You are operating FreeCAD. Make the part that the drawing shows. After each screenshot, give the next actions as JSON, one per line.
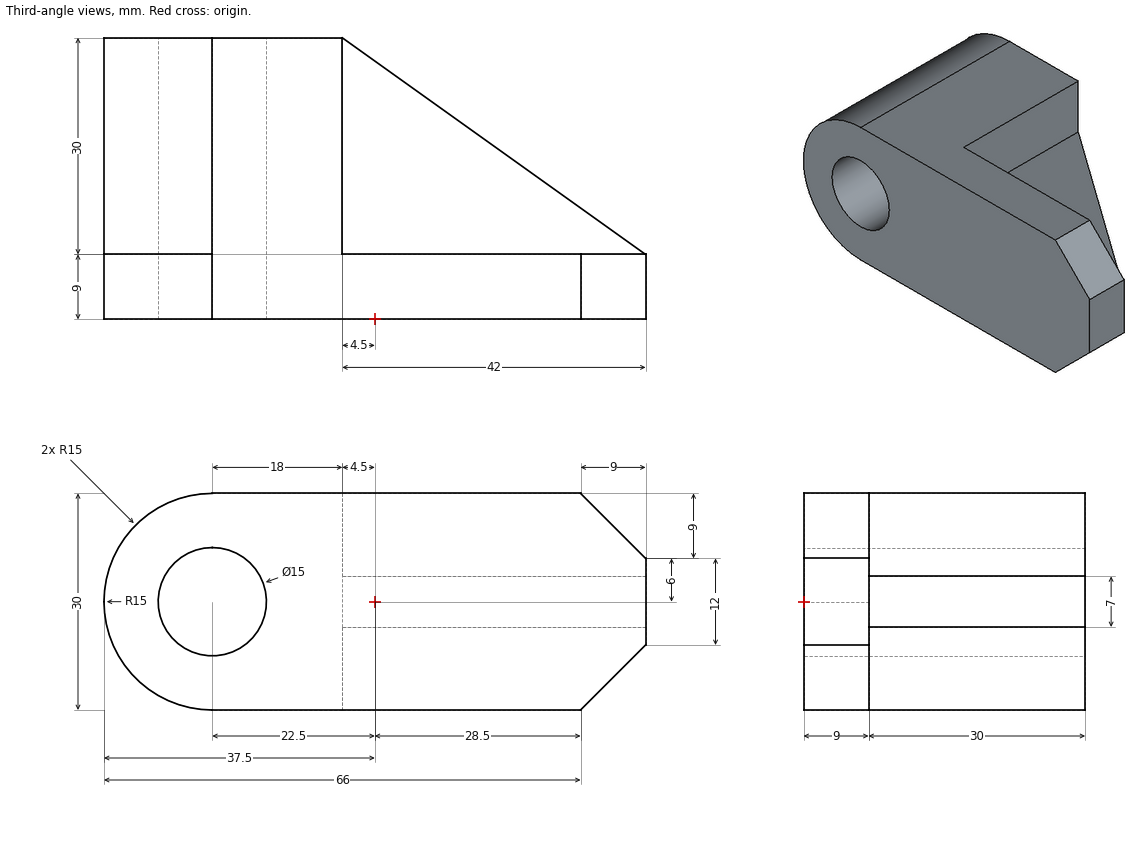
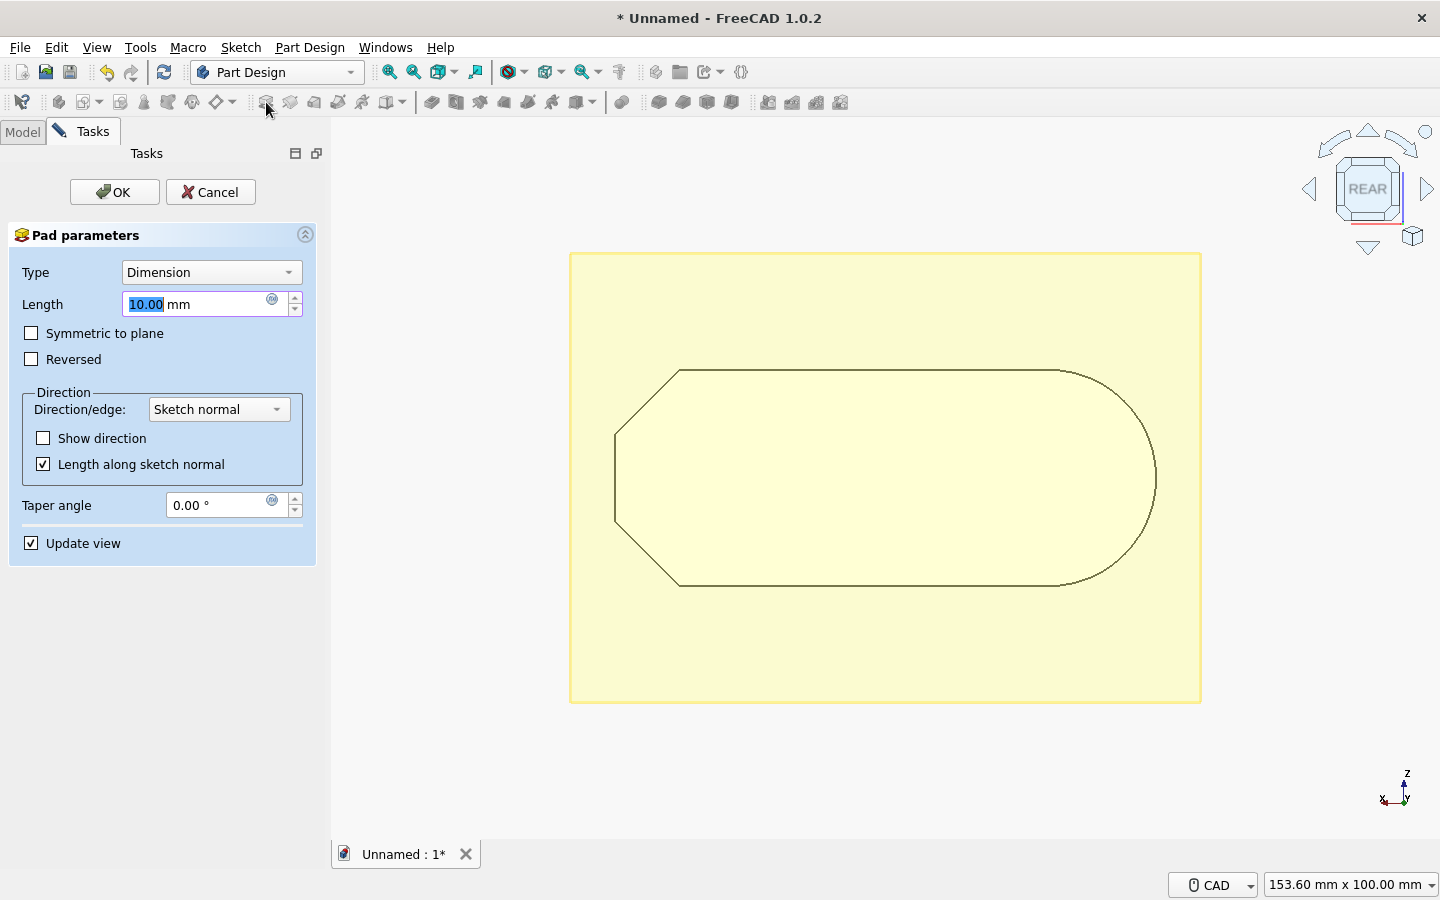
{"action": "type", "text": "30"}
{"action": "key", "text": "Tab"}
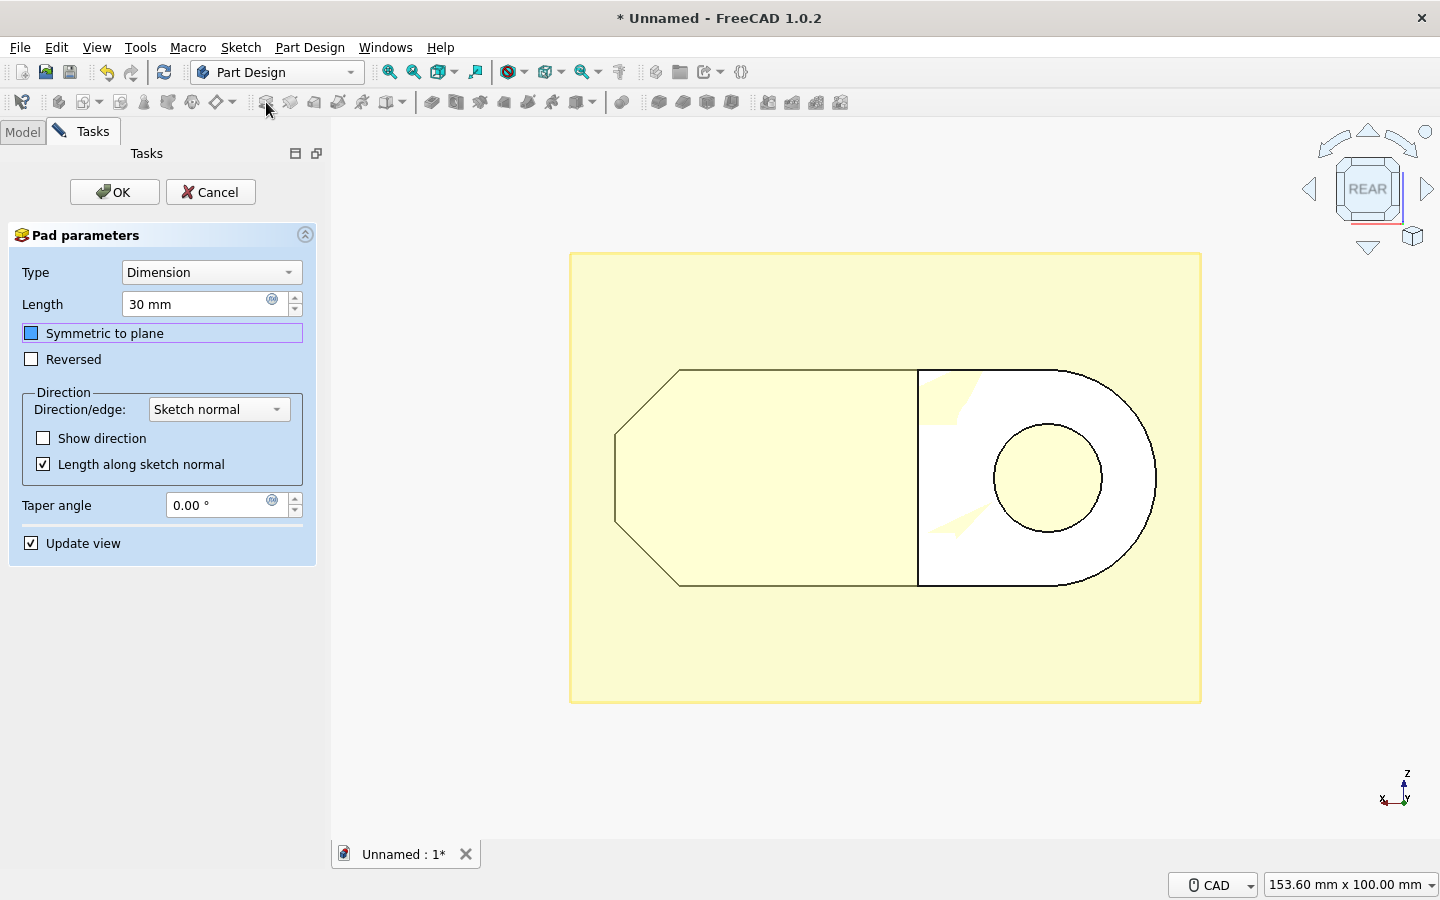
{"action": "left_click", "coordinate": [115, 192]}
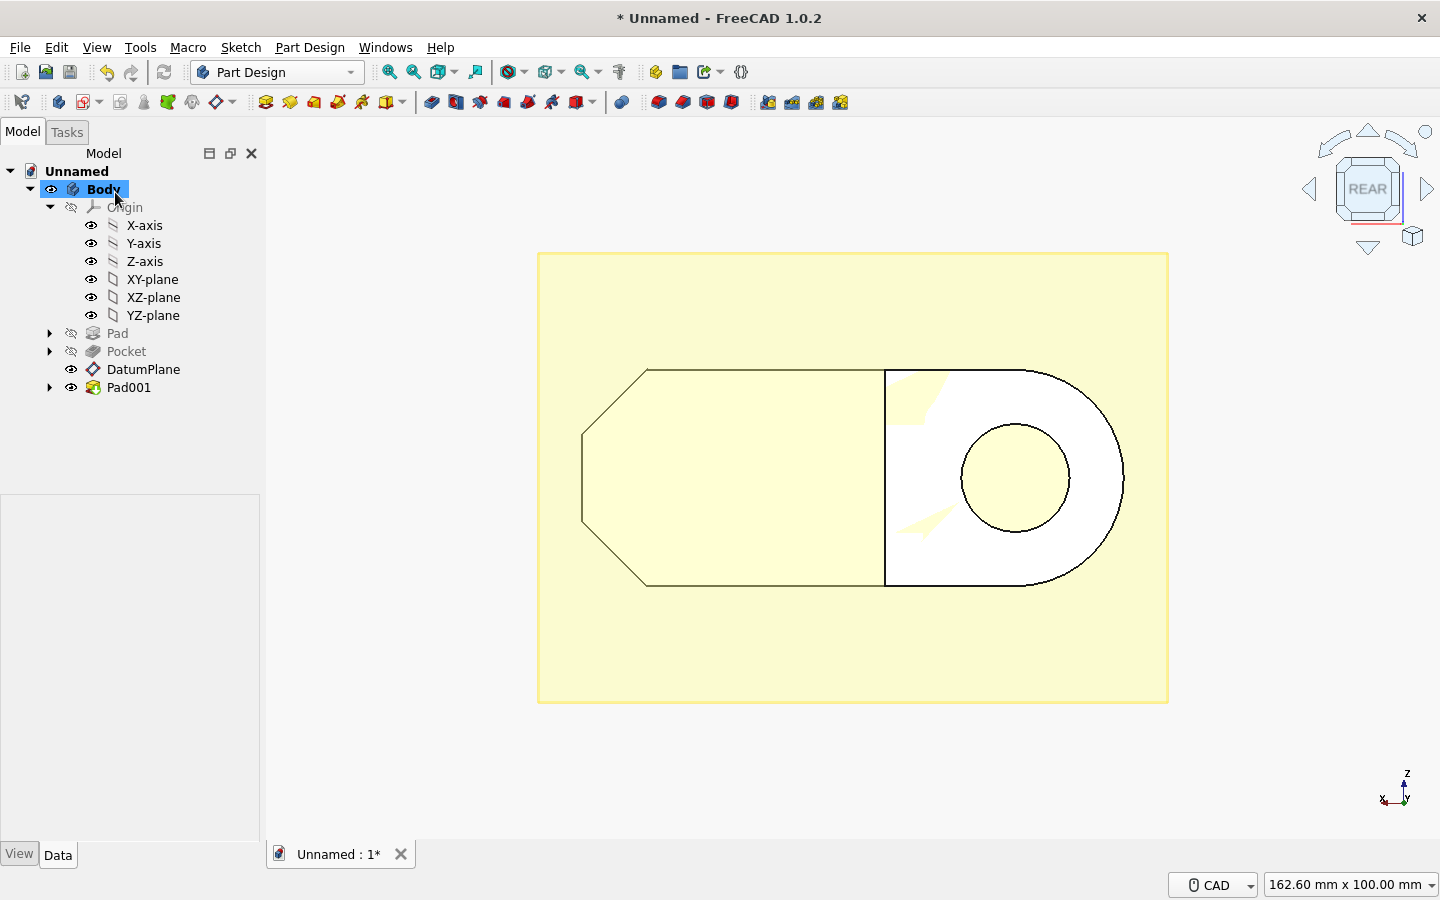
{"action": "left_click", "coordinate": [116, 369]}
{"action": "key", "text": "space"}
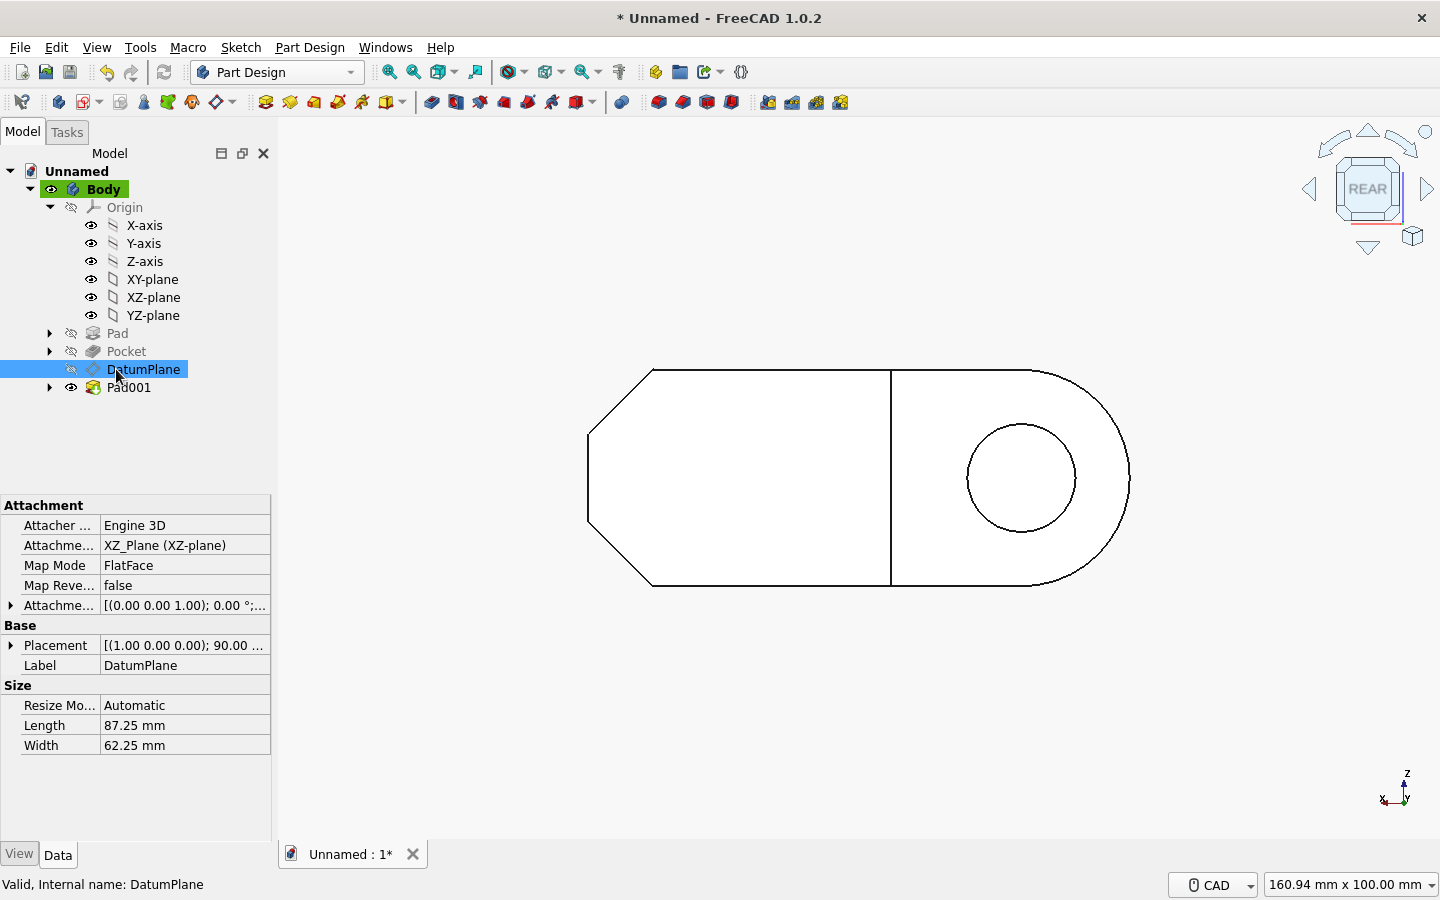
{"action": "left_click", "coordinate": [318, 799]}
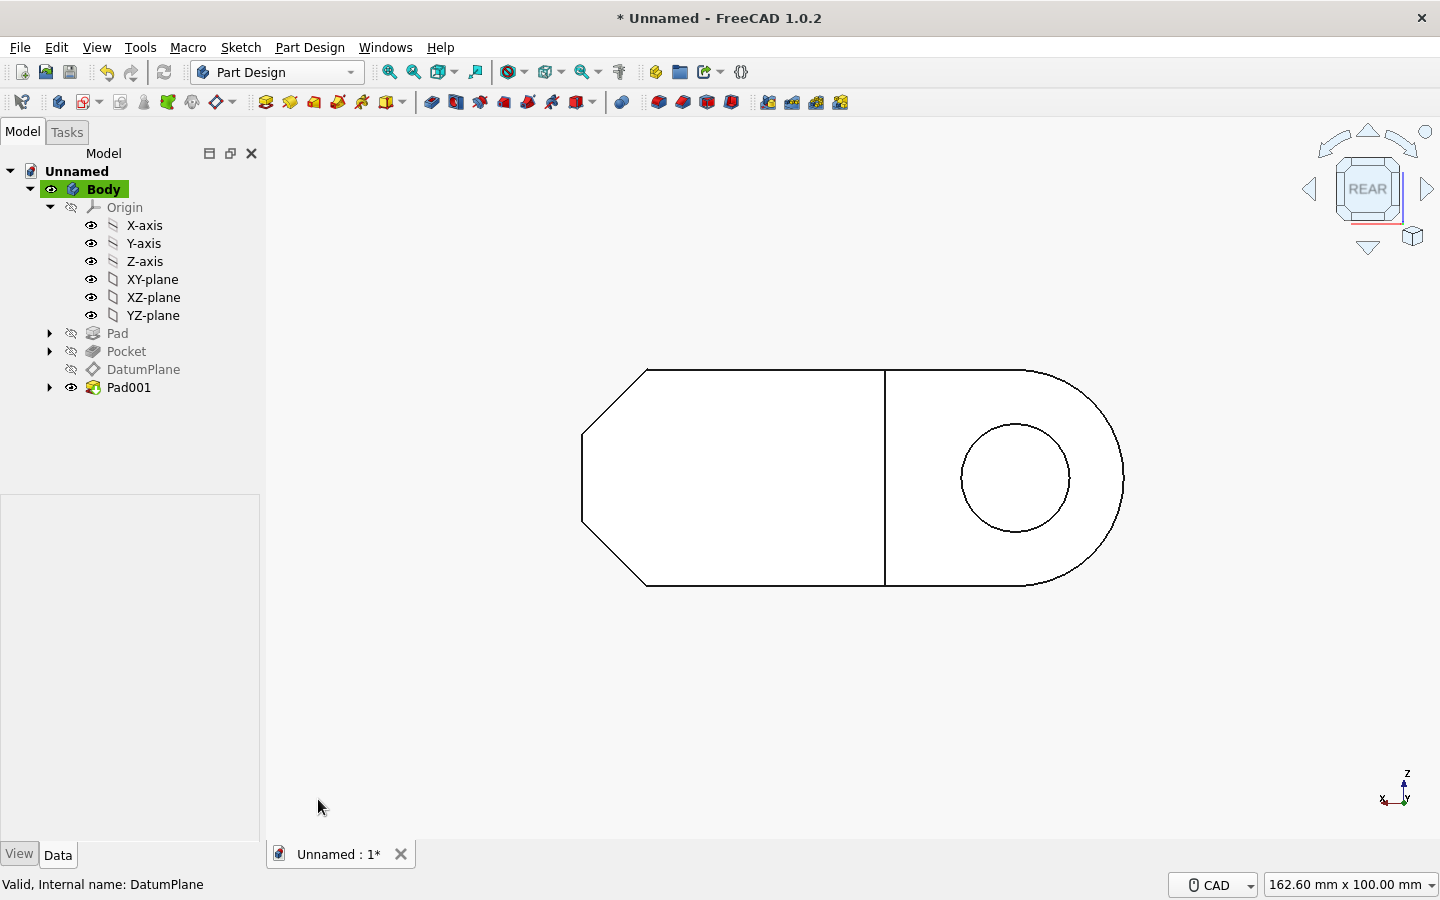
{"action": "left_click", "coordinate": [84, 102]}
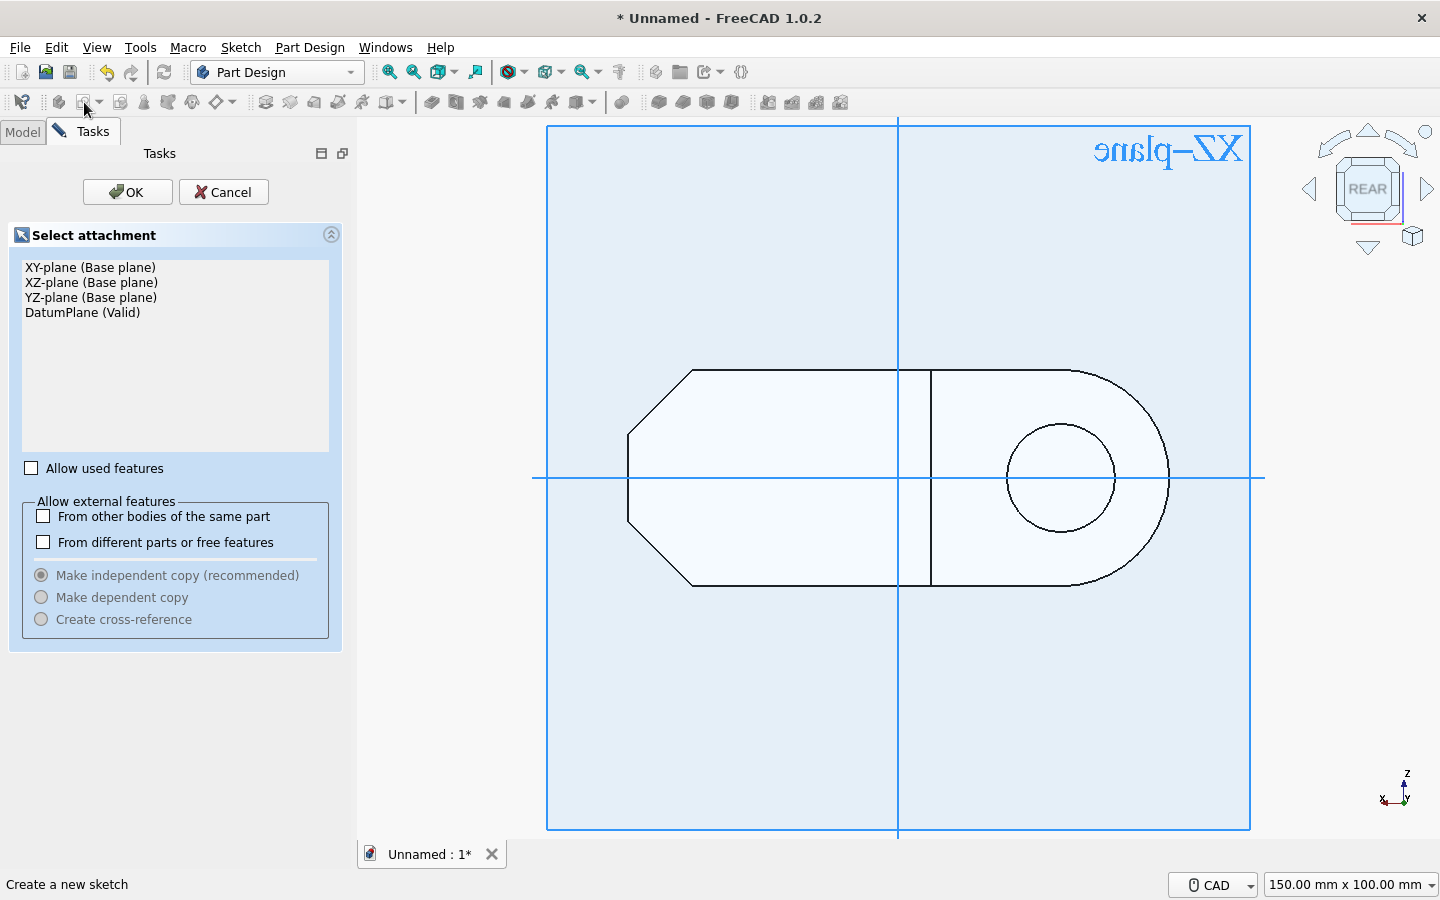
{"action": "left_click", "coordinate": [82, 268]}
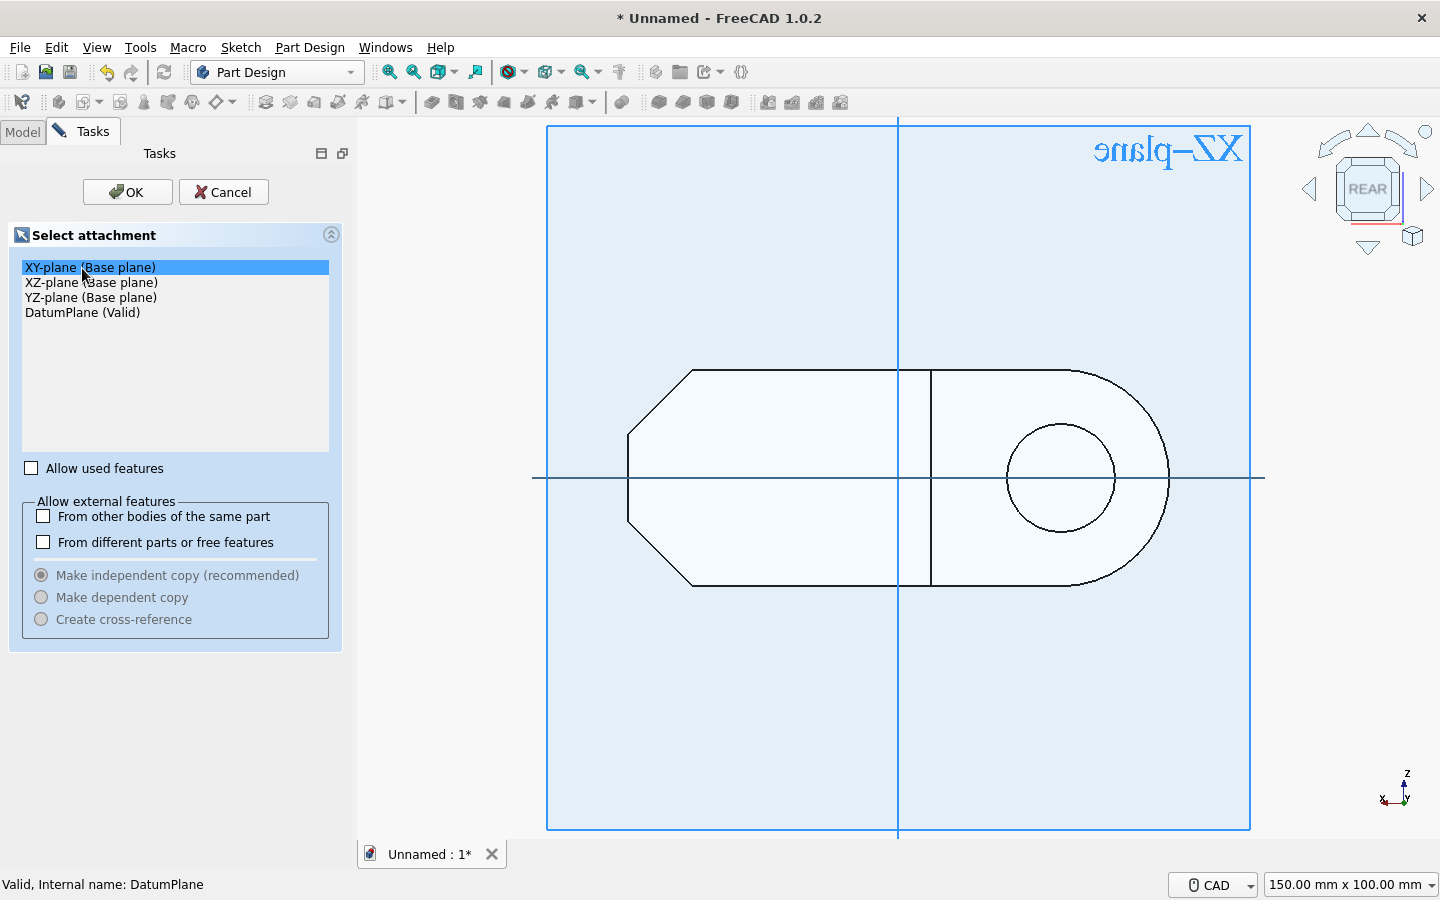
{"action": "left_click", "coordinate": [128, 192]}